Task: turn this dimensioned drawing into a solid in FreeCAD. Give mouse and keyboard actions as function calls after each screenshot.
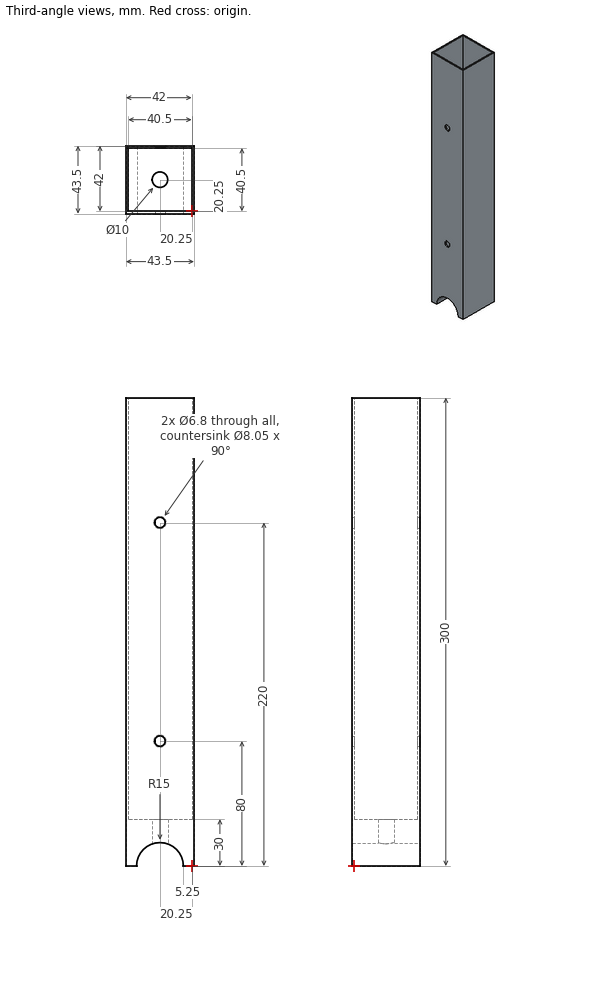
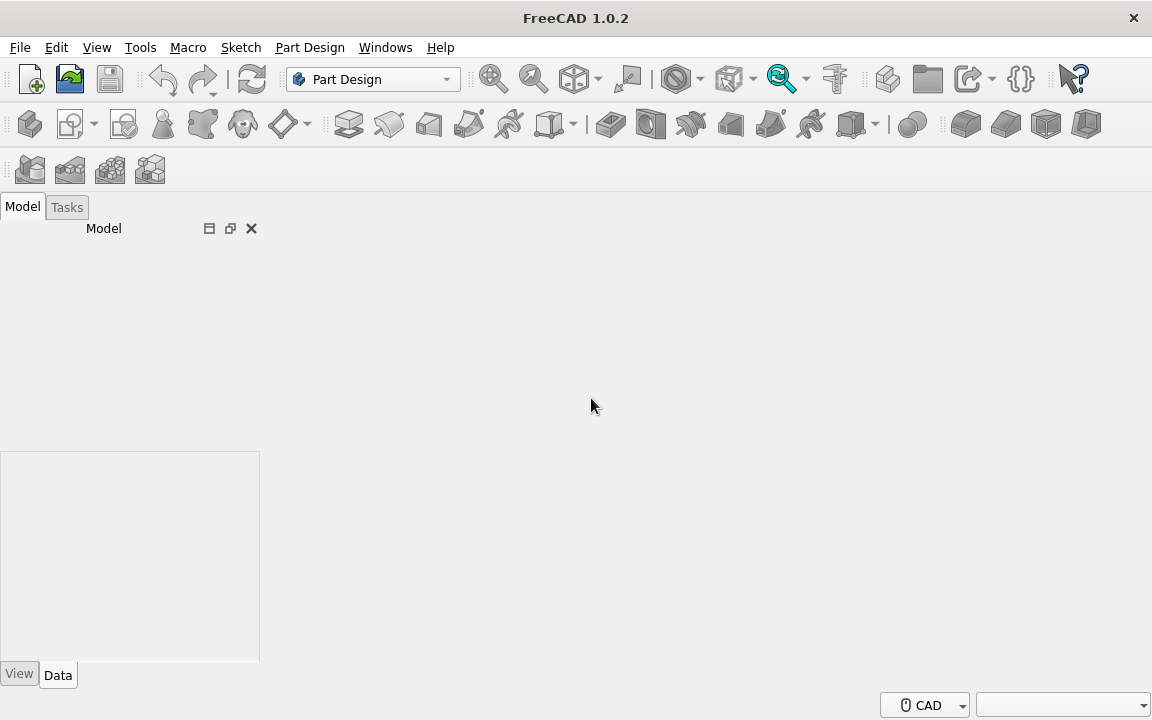
click(30, 80)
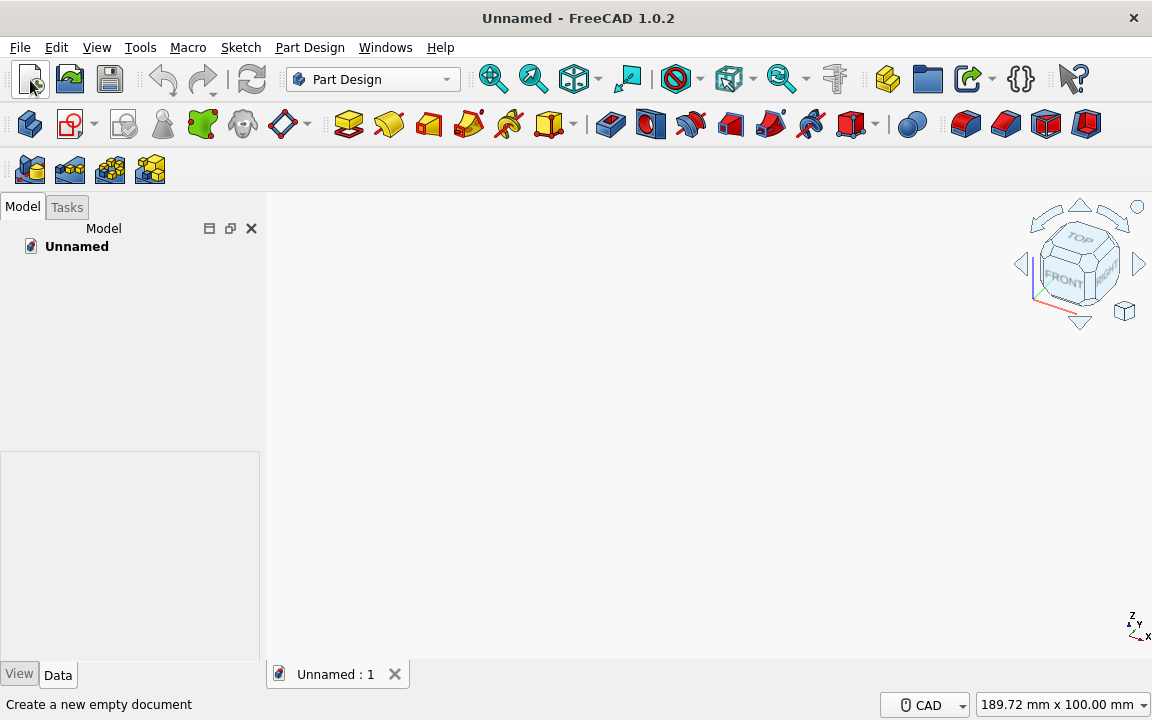
click(70, 124)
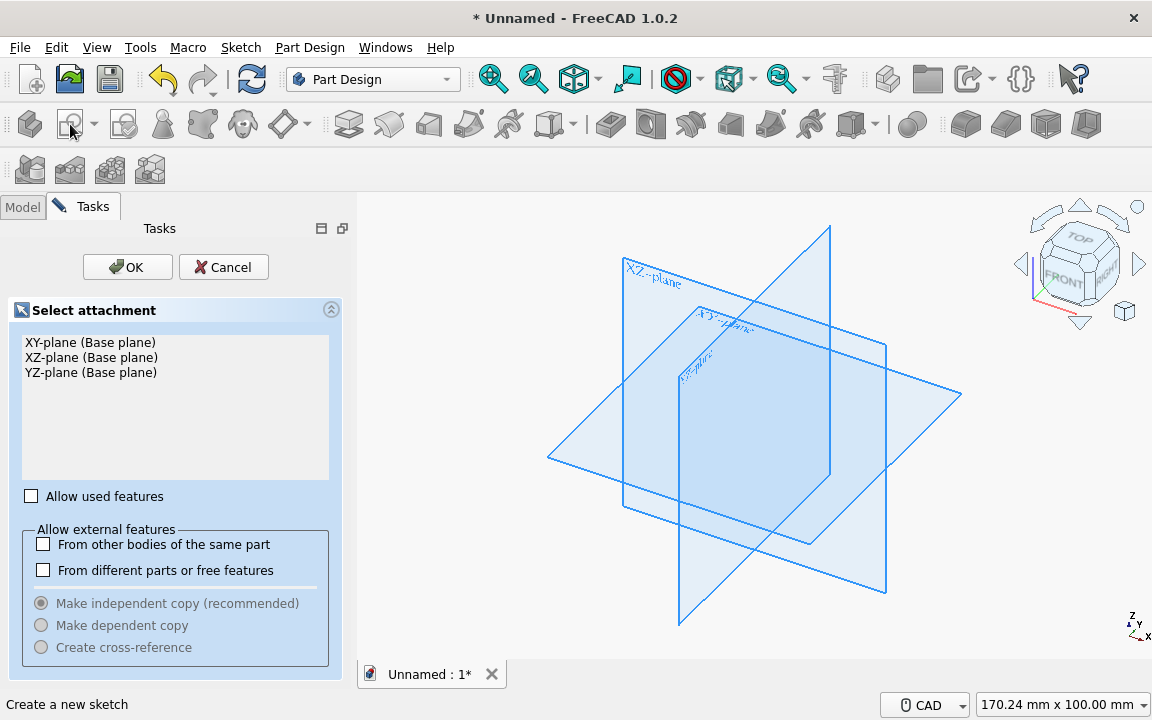
click(82, 342)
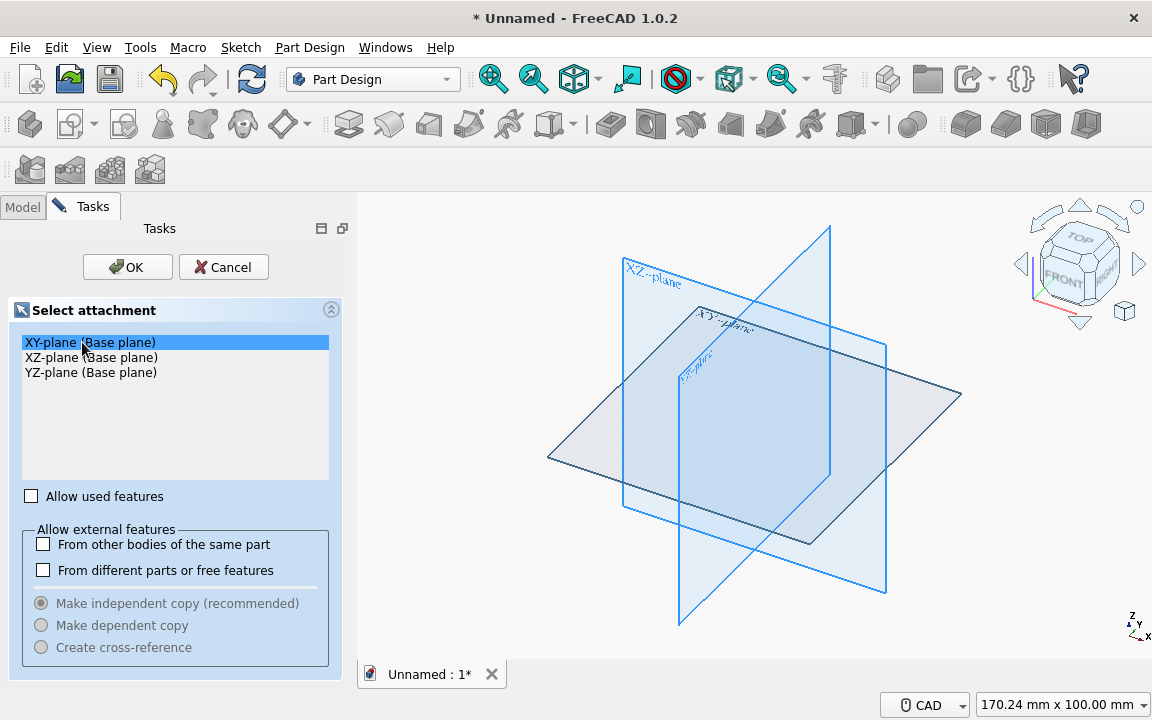
click(128, 267)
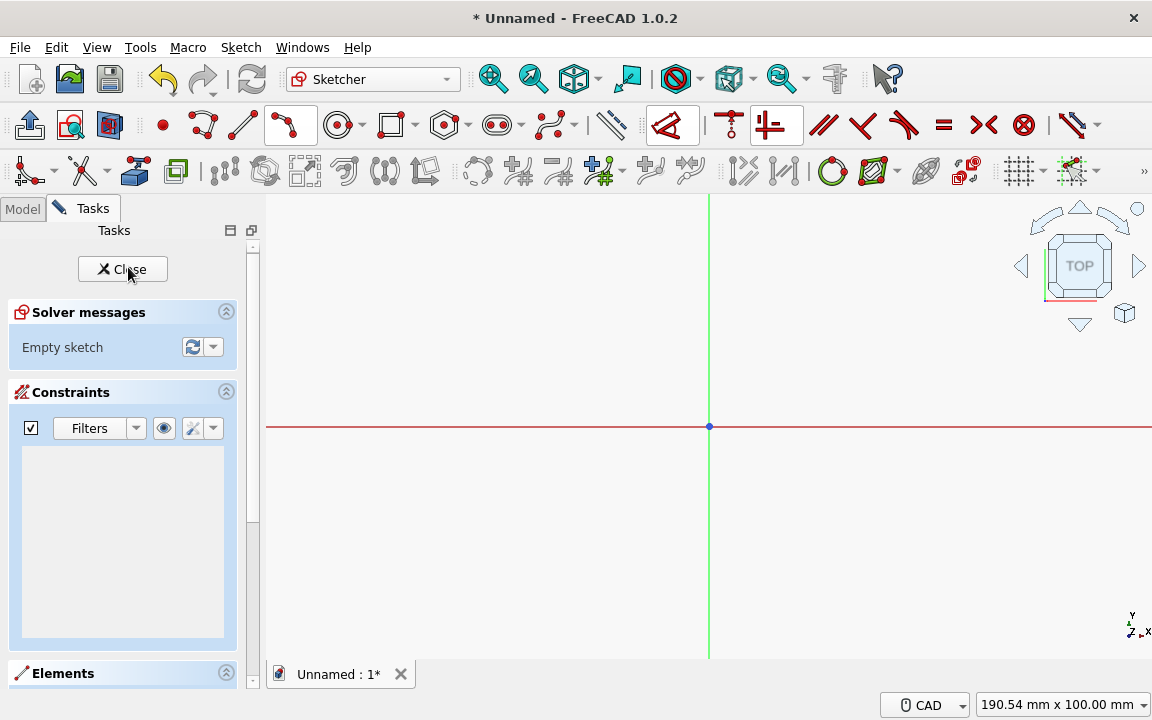
scroll(756, 631, down, 1)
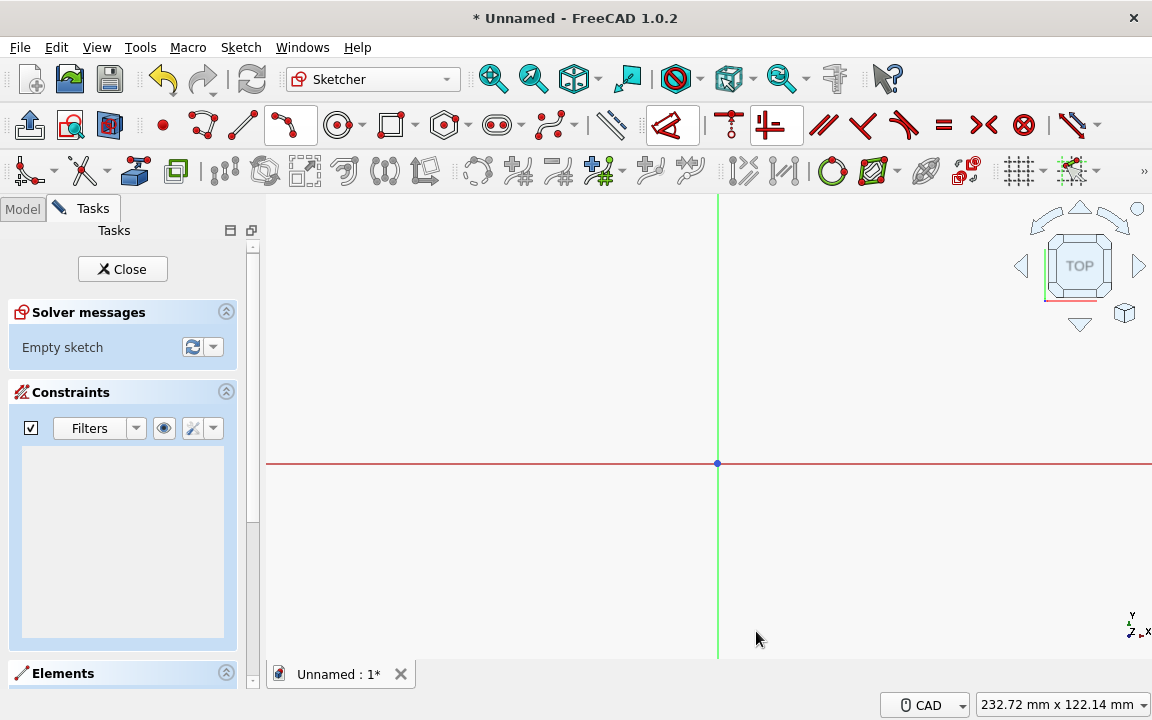
scroll(641, 338, up, 3)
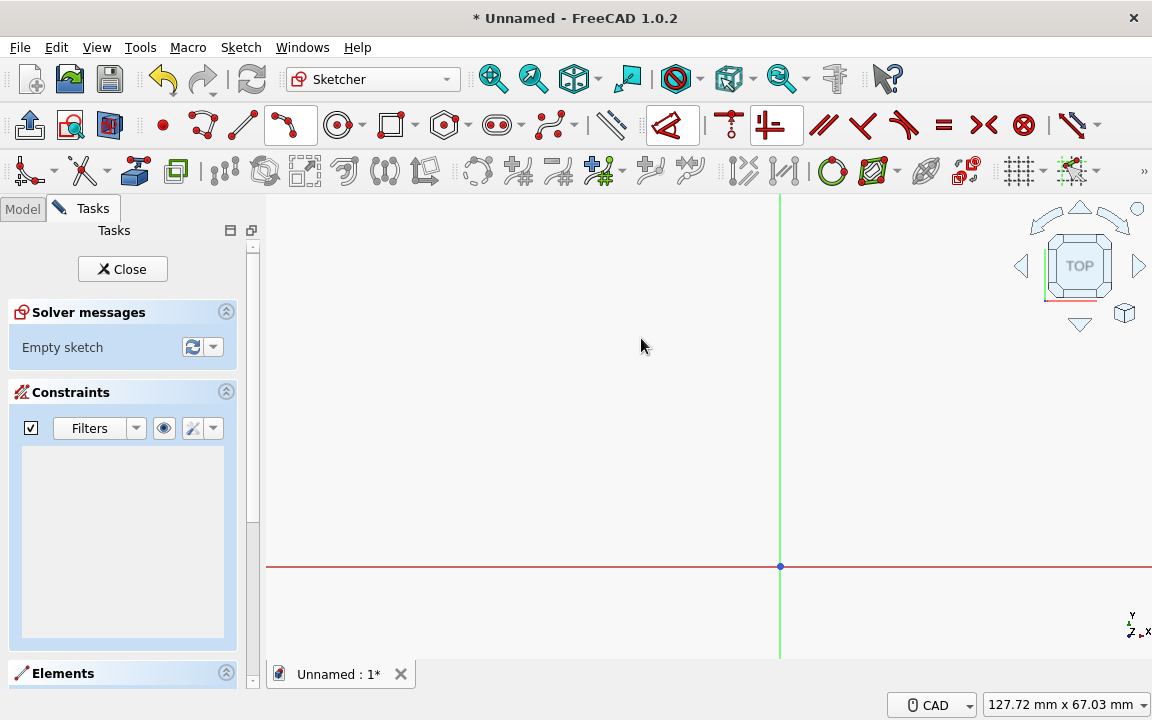
click(392, 126)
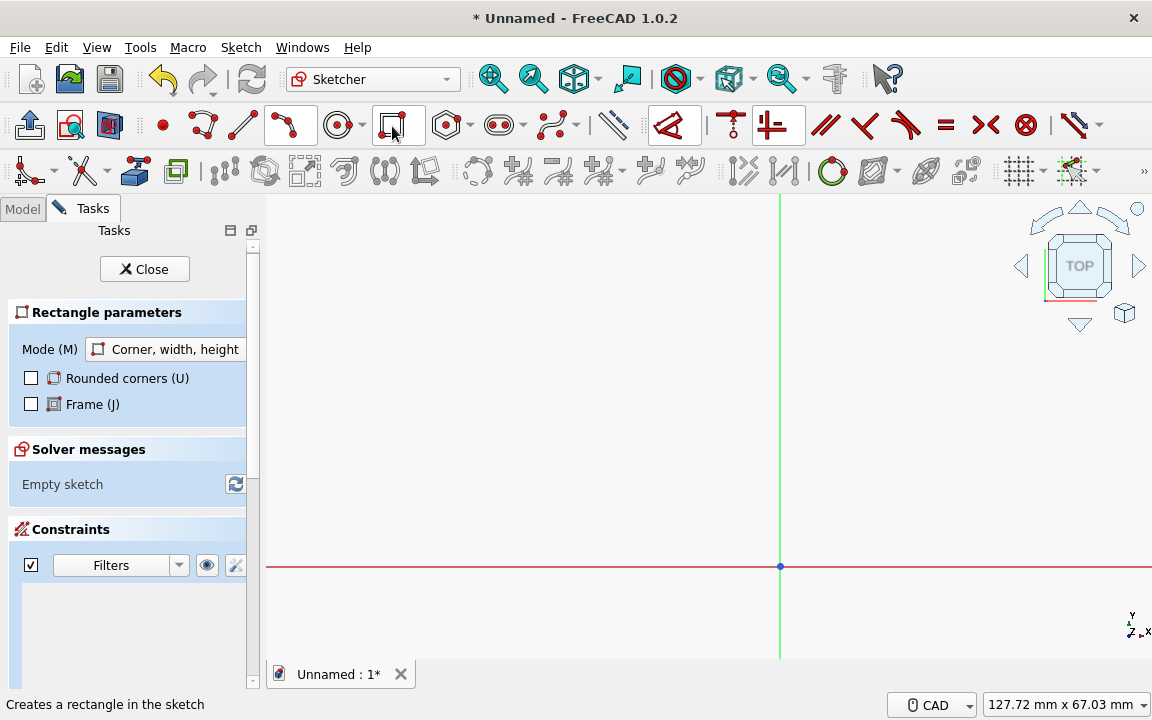
click(489, 276)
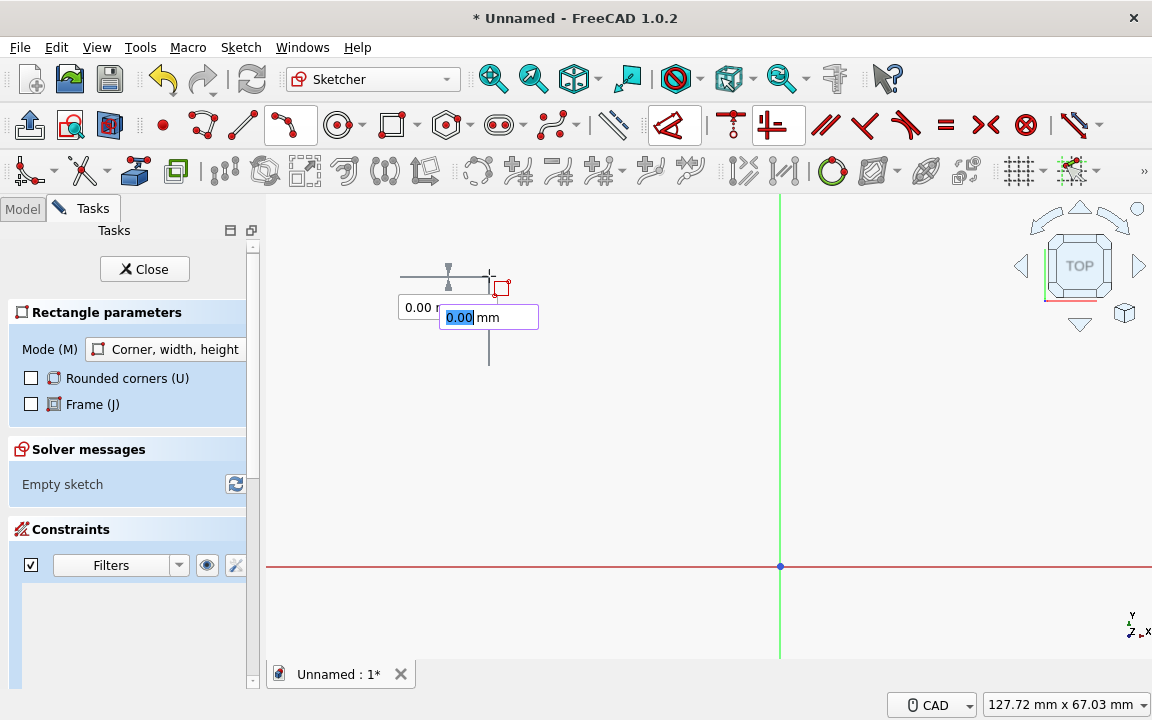
scroll(791, 577, up, 3)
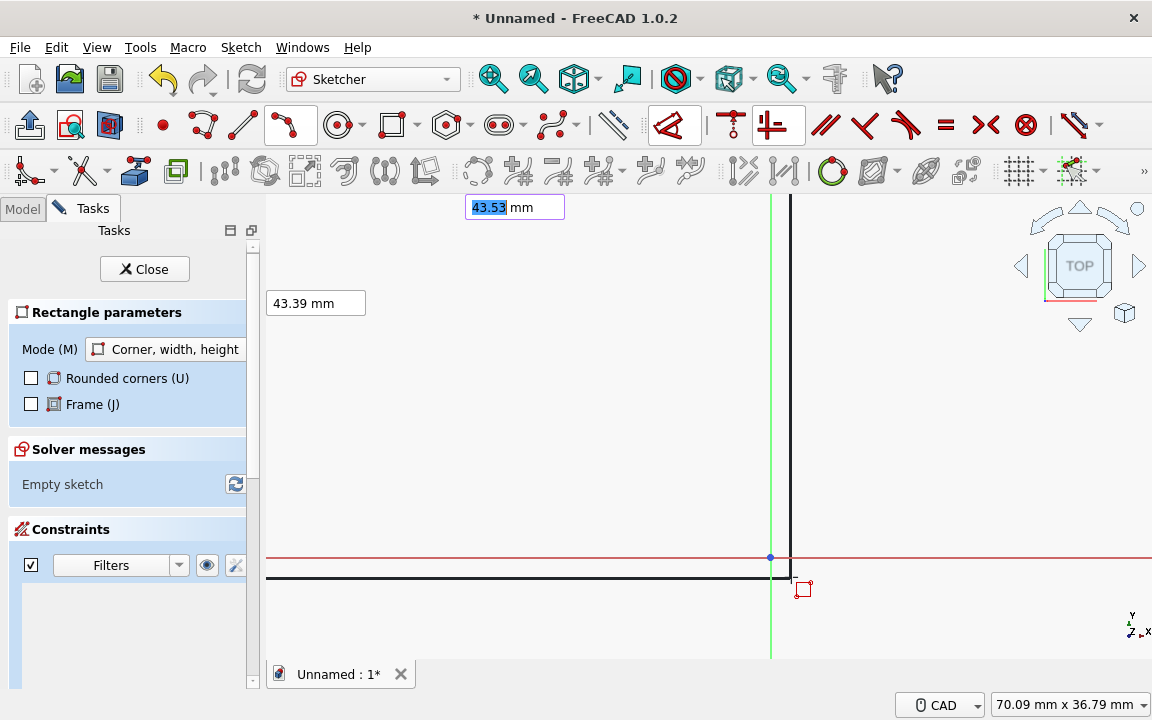
click(790, 577)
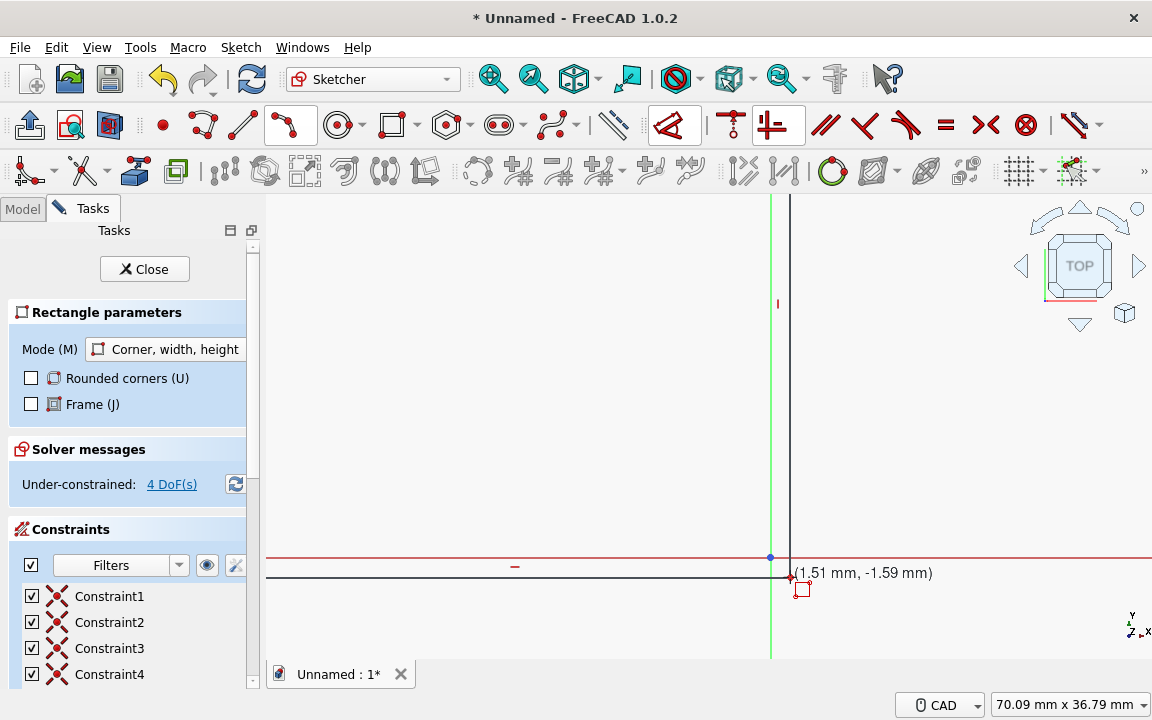
click(771, 558)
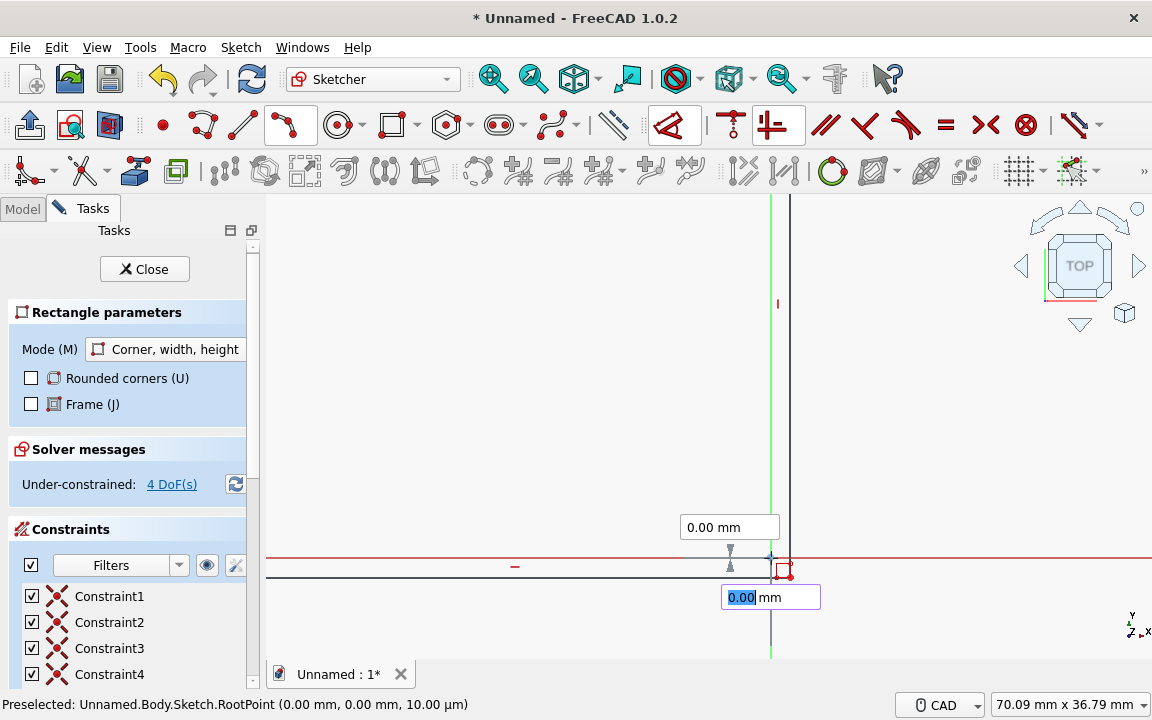
scroll(793, 578, down, 3)